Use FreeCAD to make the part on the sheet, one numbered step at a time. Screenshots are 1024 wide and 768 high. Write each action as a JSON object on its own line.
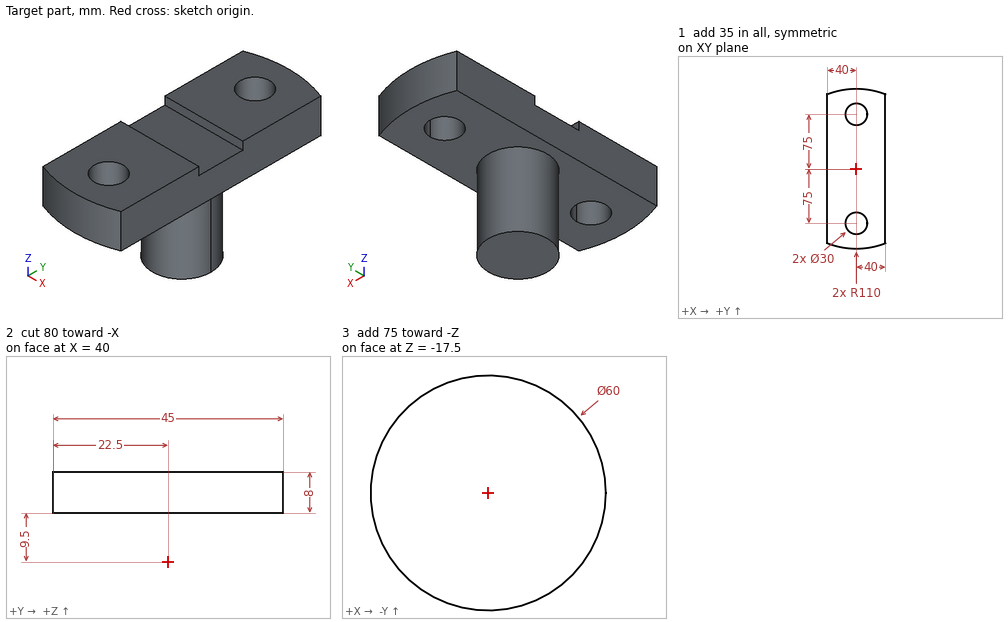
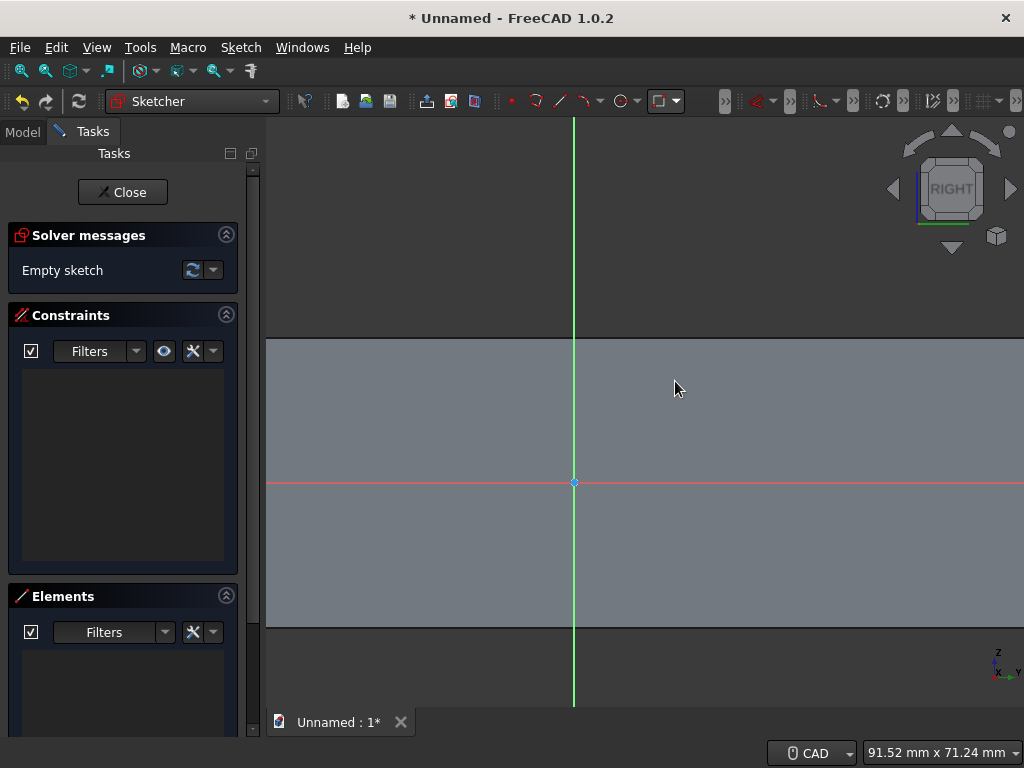
{"action": "key", "text": "g r"}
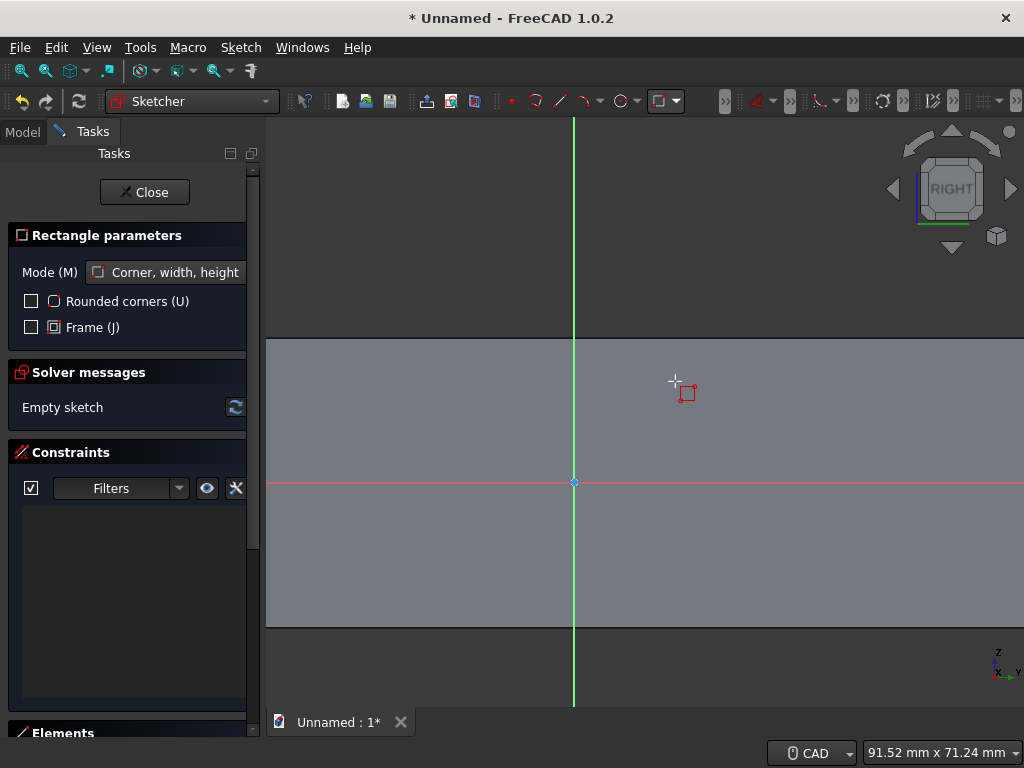
{"action": "left_click", "coordinate": [388, 338]}
{"action": "mouse_move", "coordinate": [760, 404]}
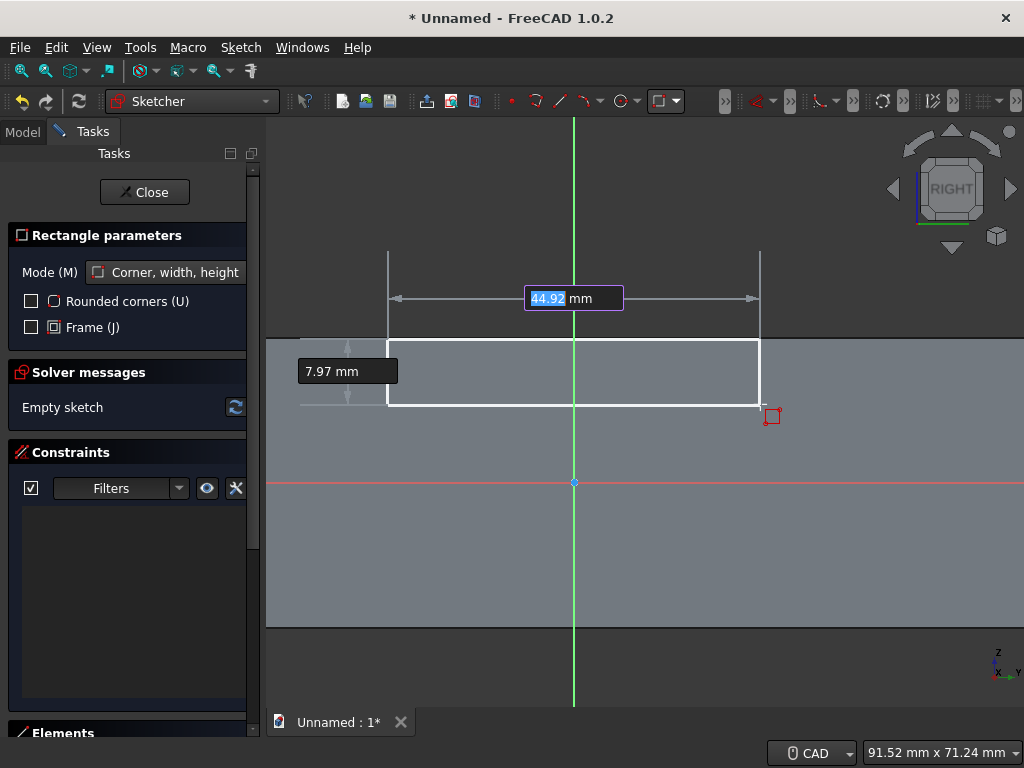
{"action": "type", "text": "45"}
{"action": "key", "text": "Tab"}
{"action": "type", "text": "8"}
{"action": "key", "text": "Return"}
{"action": "key", "text": "Escape"}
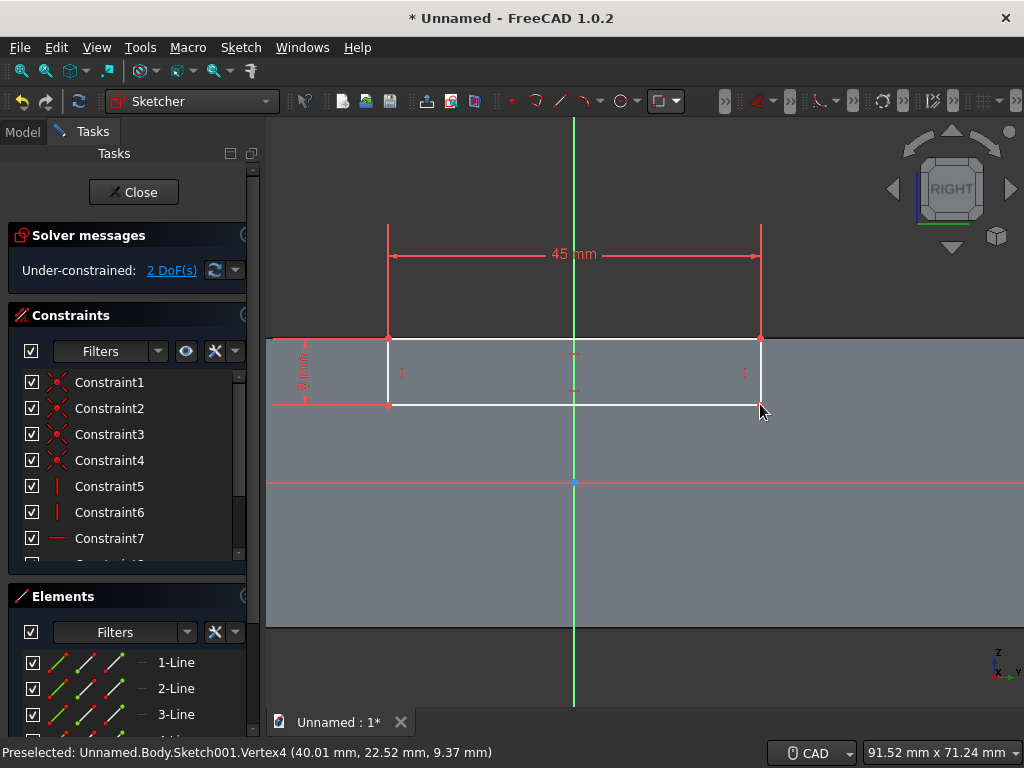
{"action": "key", "text": "d"}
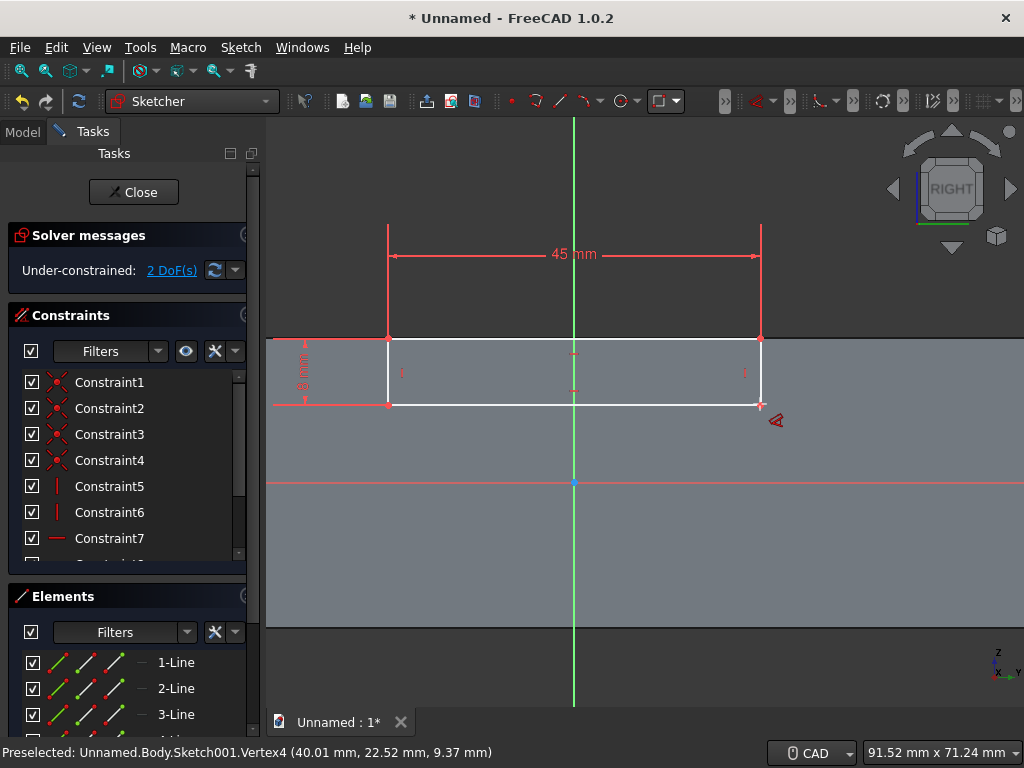
{"action": "left_click", "coordinate": [388, 405]}
{"action": "left_click", "coordinate": [354, 444]}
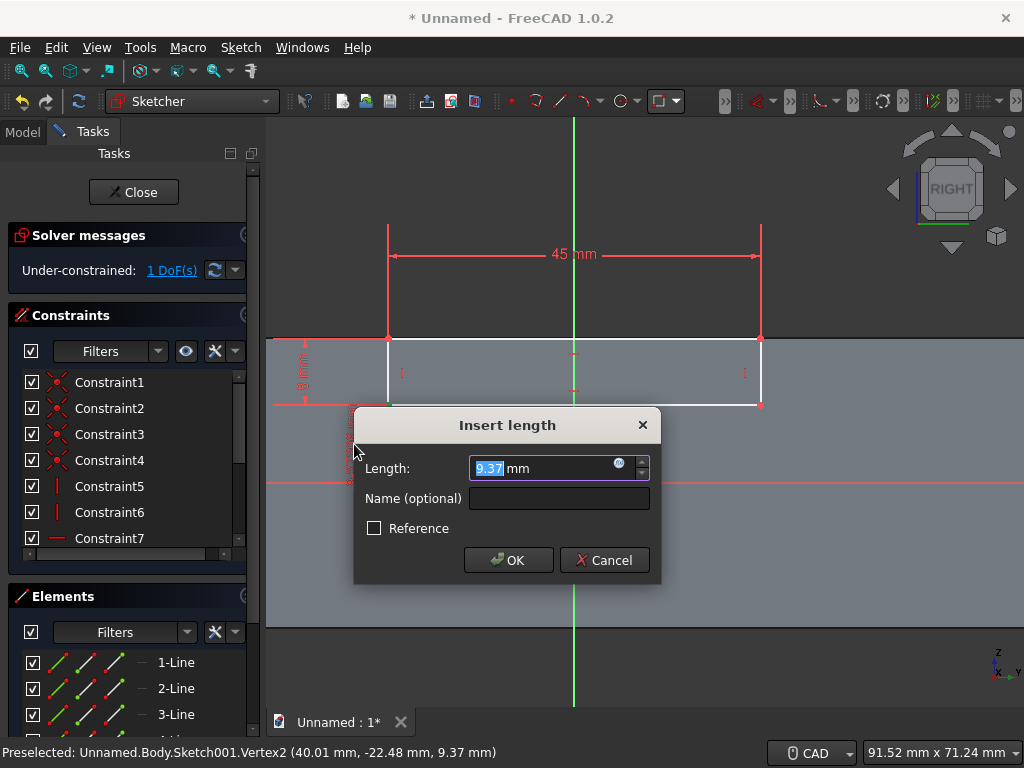
{"action": "type", "text": "9.5"}
{"action": "key", "text": "Return"}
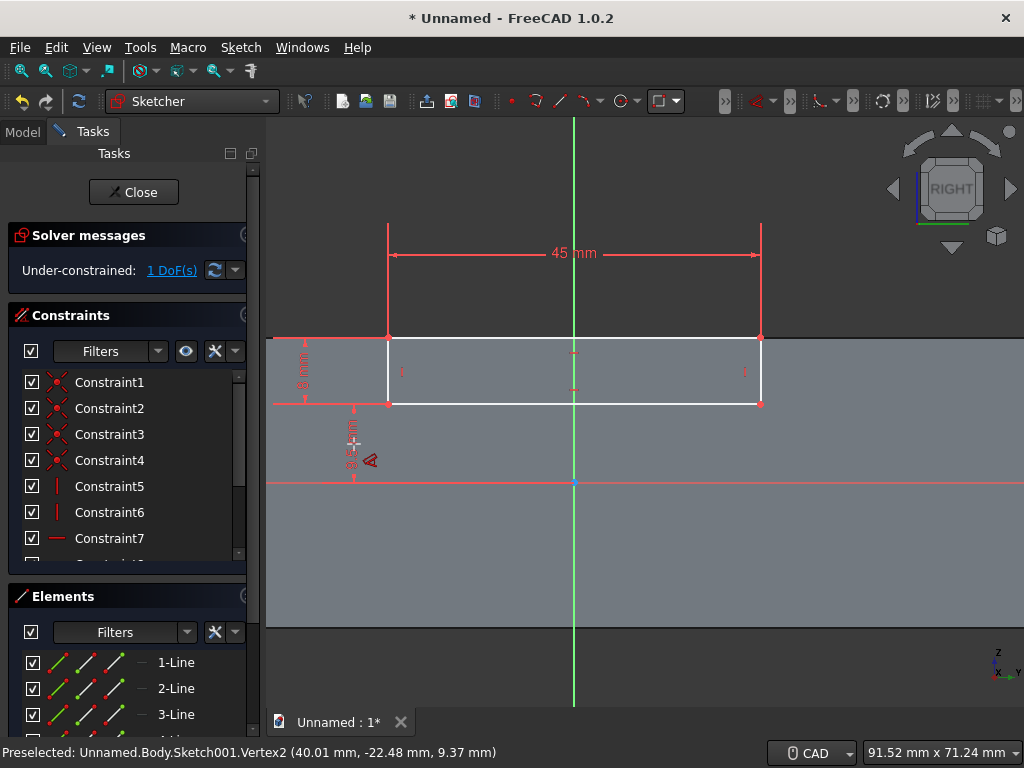
{"action": "left_click", "coordinate": [388, 338]}
{"action": "left_click", "coordinate": [481, 517]}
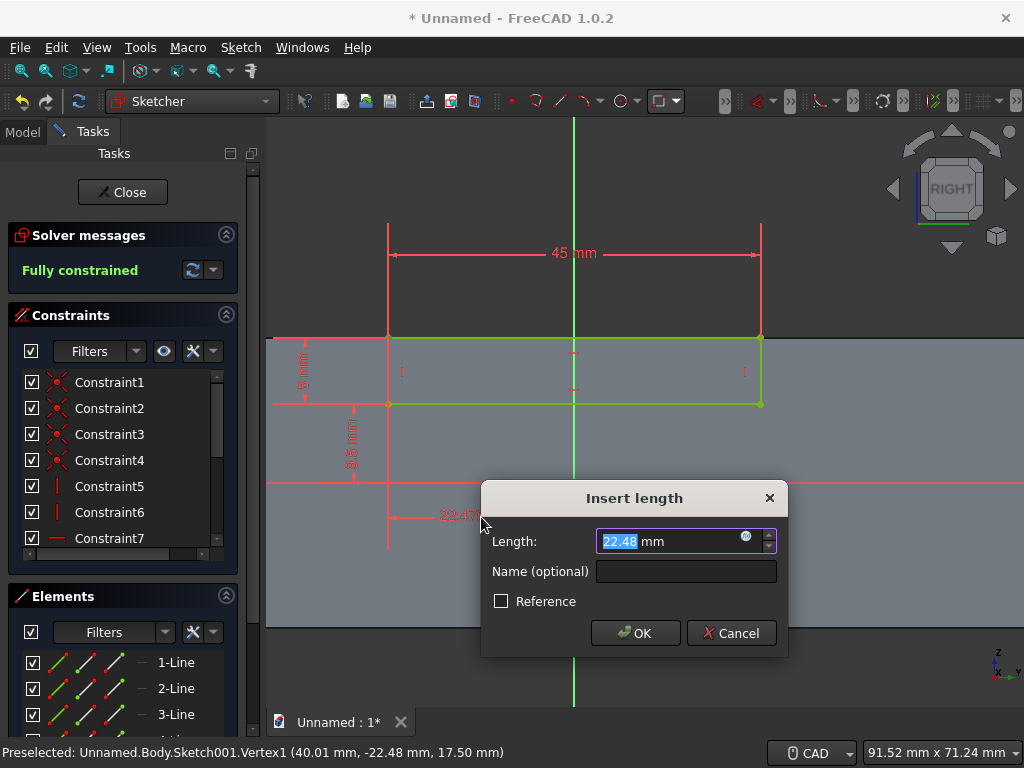
{"action": "type", "text": "22.5"}
{"action": "key", "text": "Return"}
{"action": "key", "text": "Escape"}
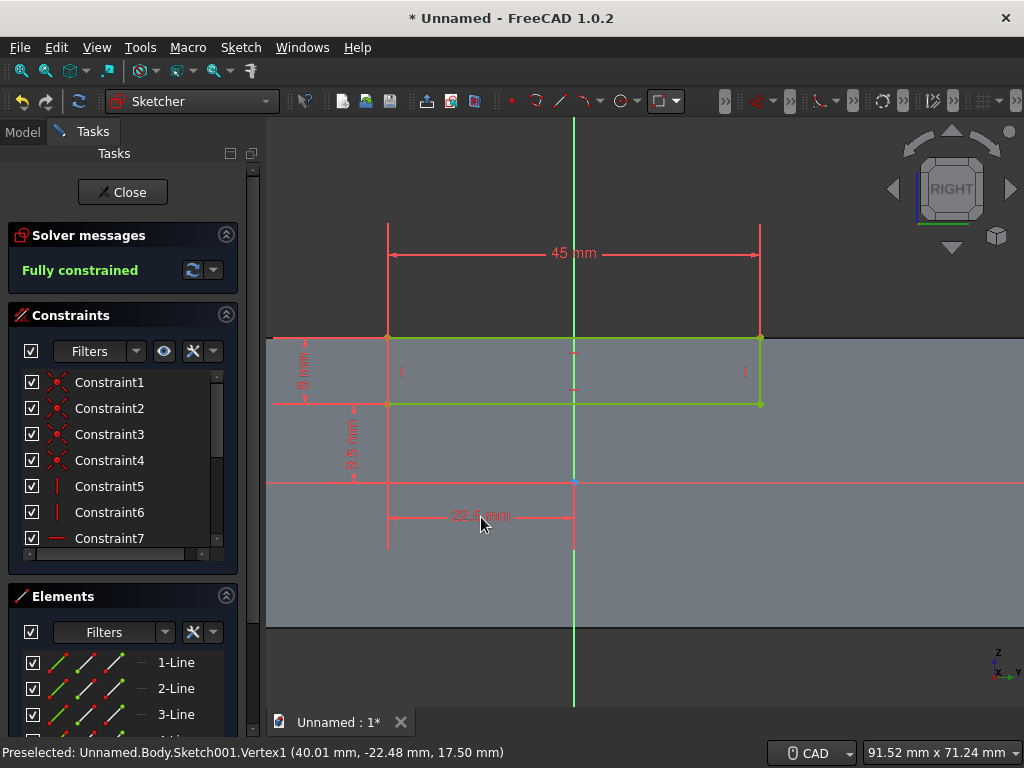
{"action": "left_click", "coordinate": [123, 192]}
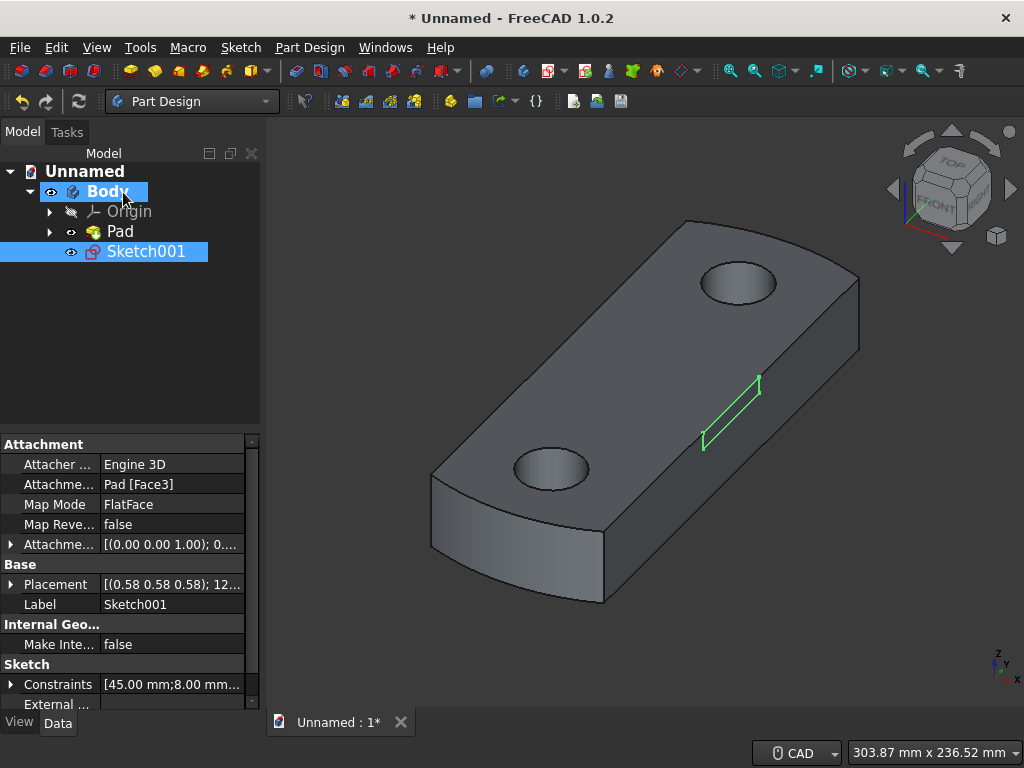
{"action": "left_click", "coordinate": [298, 72]}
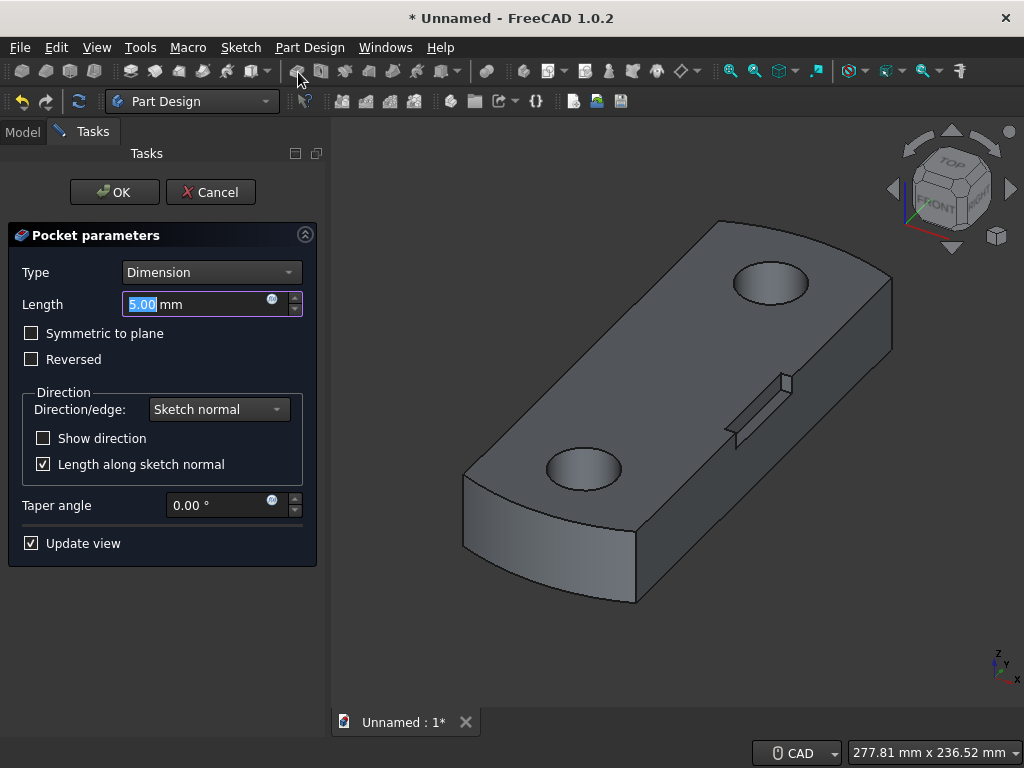
{"action": "type", "text": "80"}
{"action": "key", "text": "Tab"}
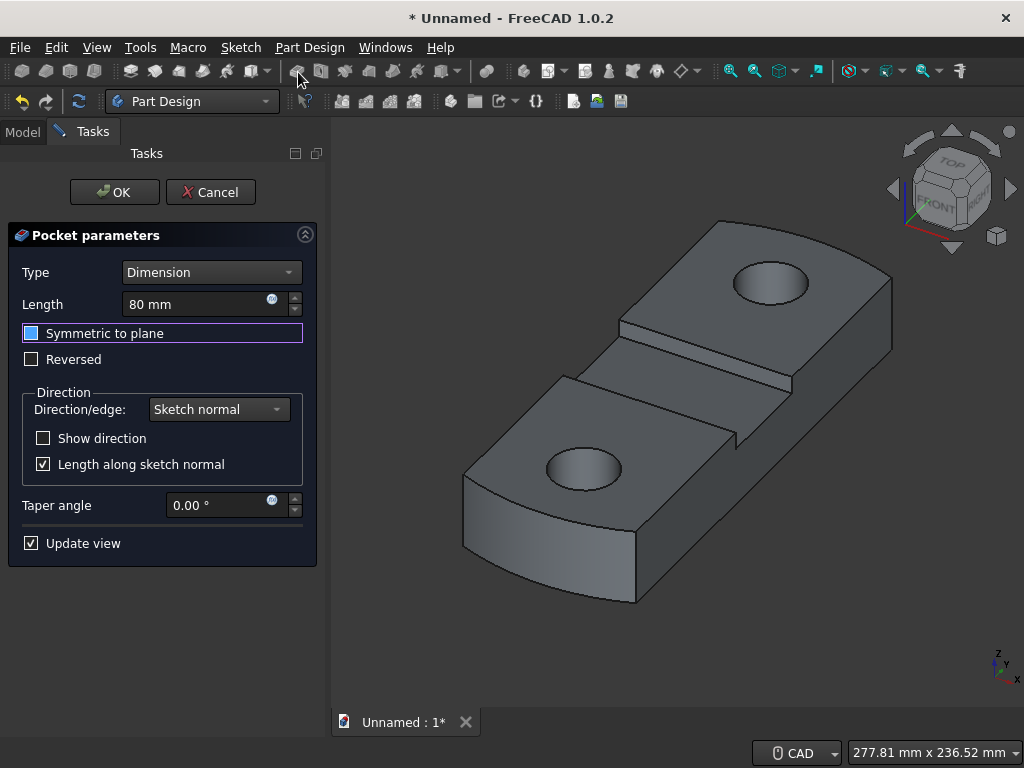
{"action": "left_click", "coordinate": [115, 192]}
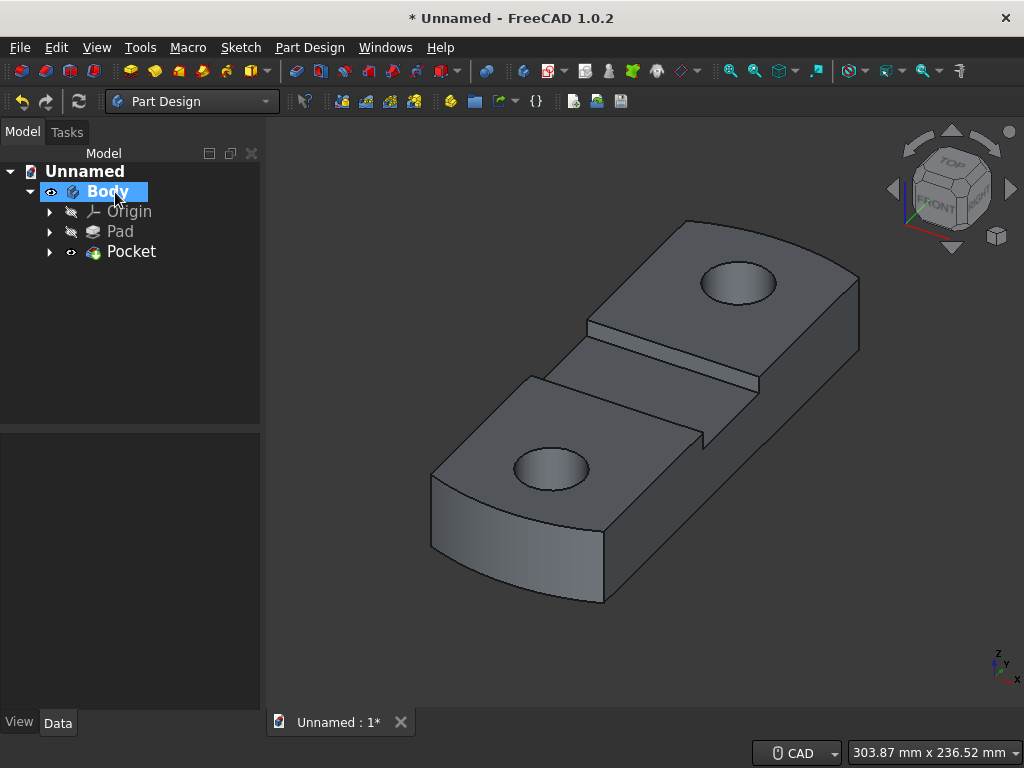
{"action": "key", "text": "5"}